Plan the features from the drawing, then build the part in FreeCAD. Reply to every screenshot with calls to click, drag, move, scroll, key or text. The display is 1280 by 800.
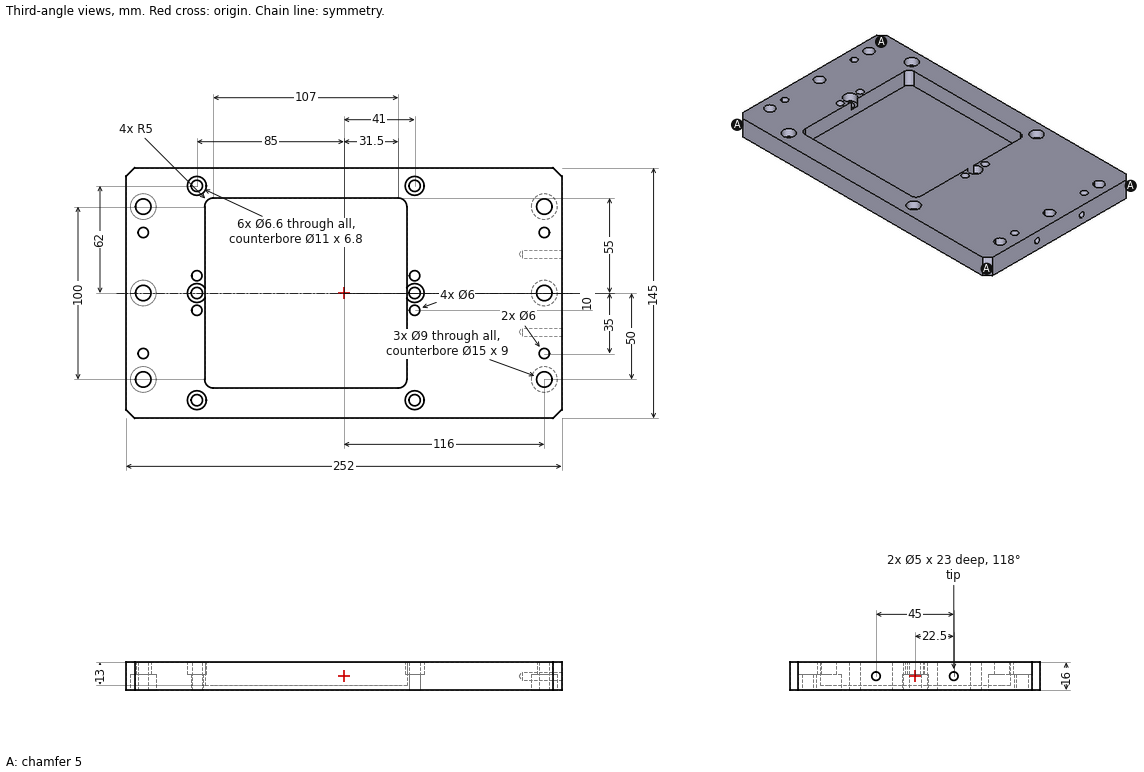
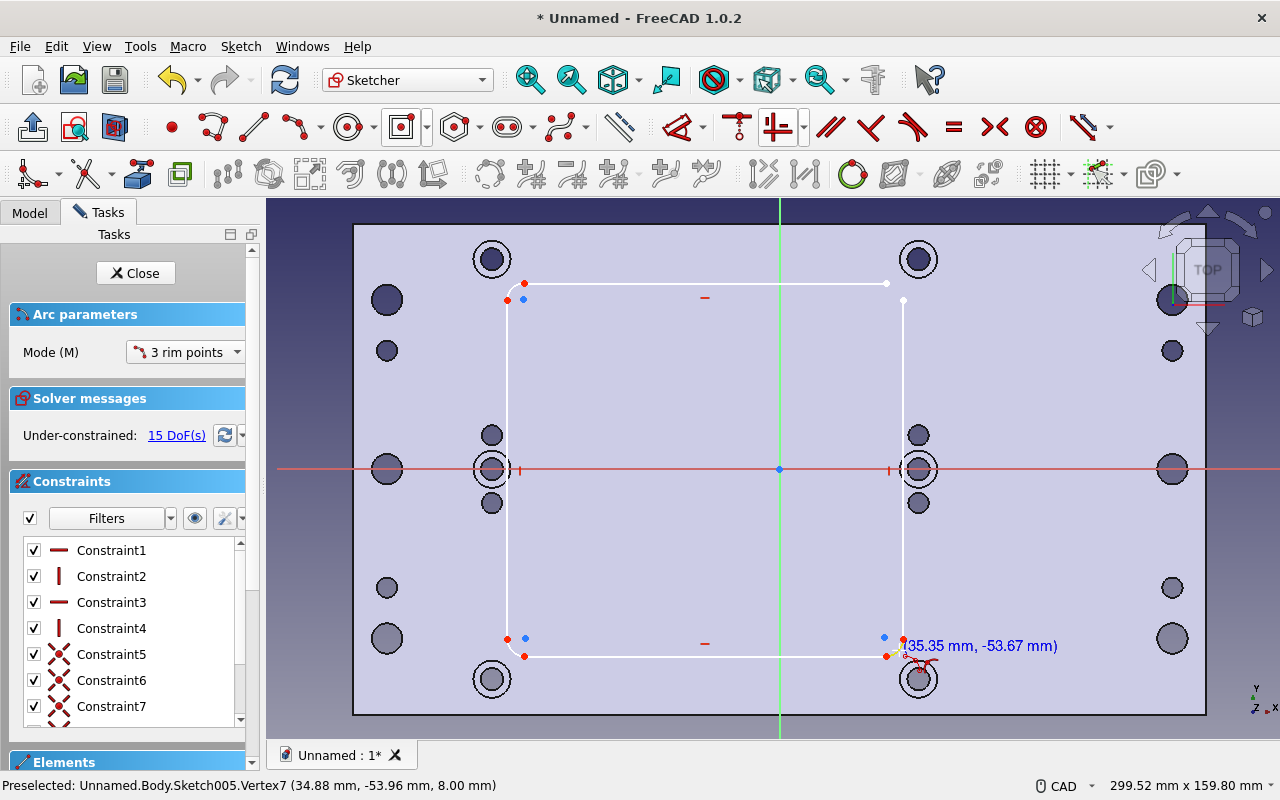
click(903, 301)
click(886, 284)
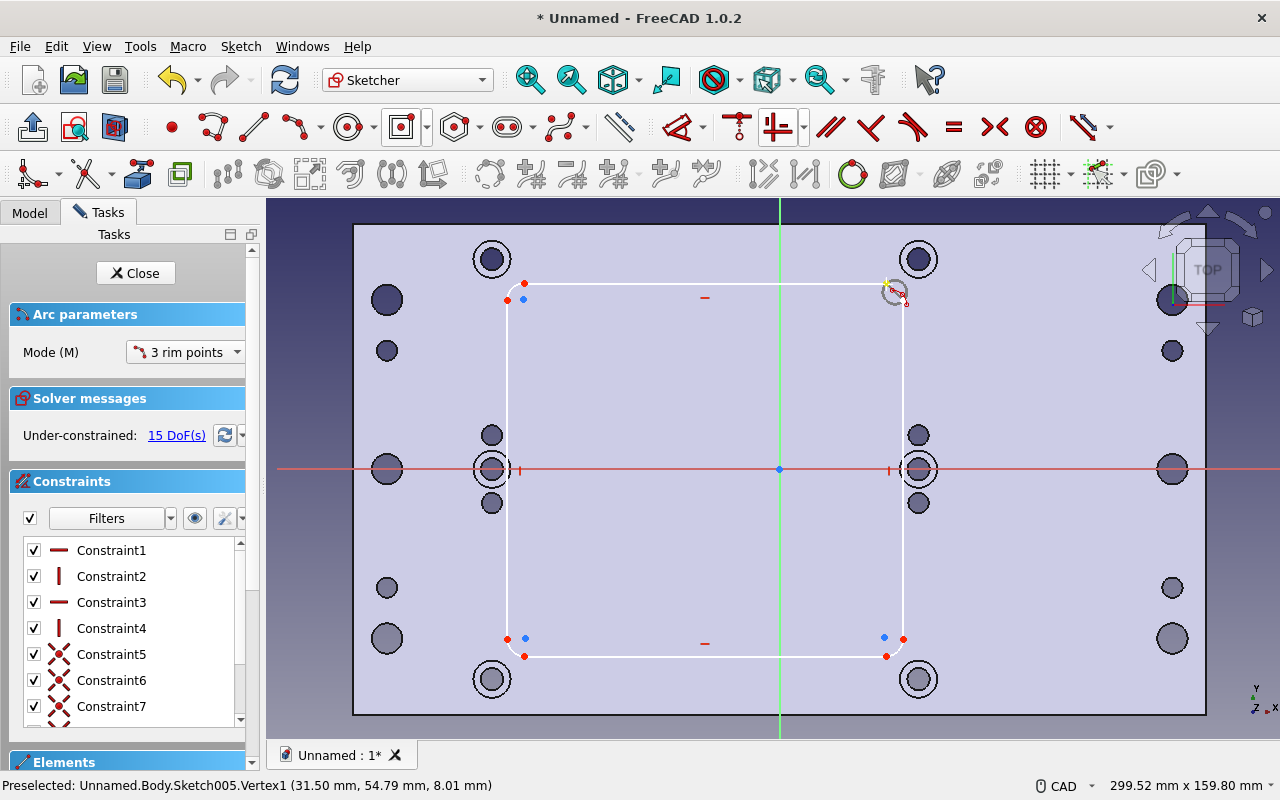
scroll(898, 288, up, 6)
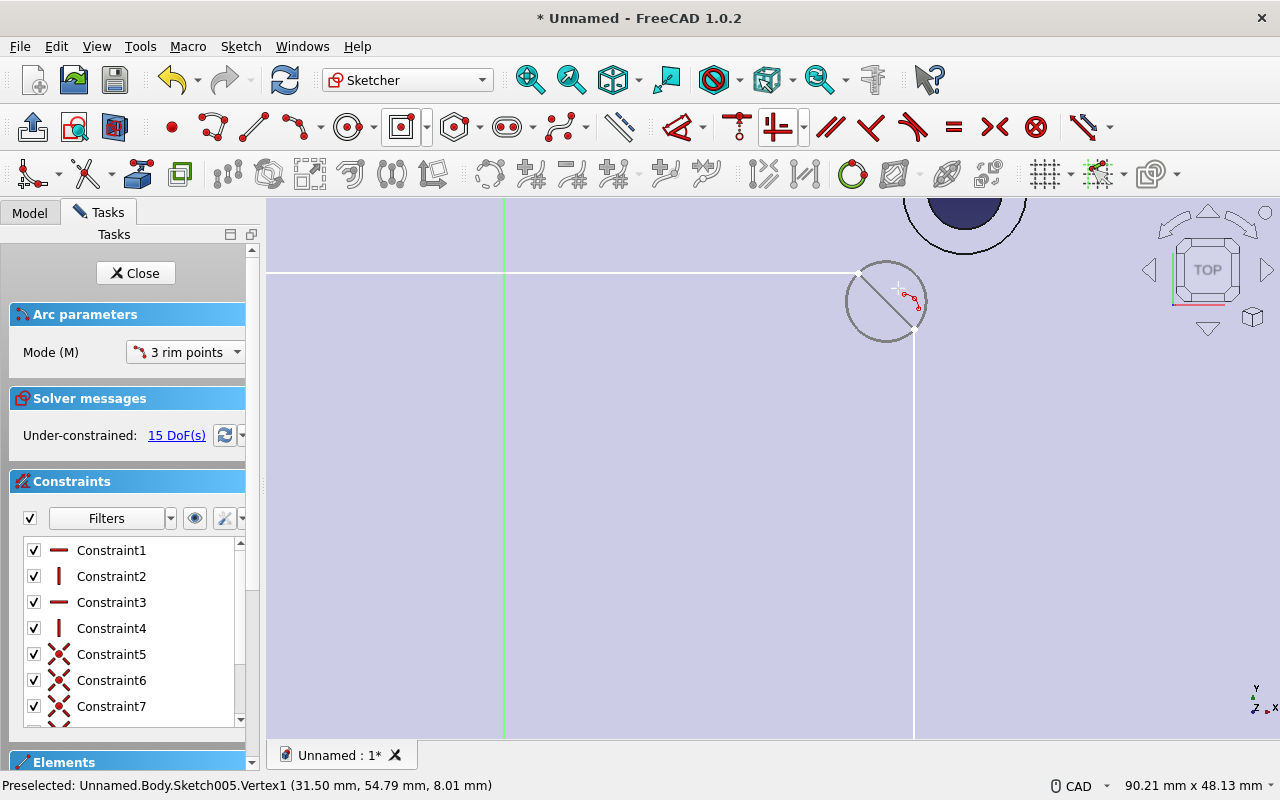
click(898, 287)
key(Escape)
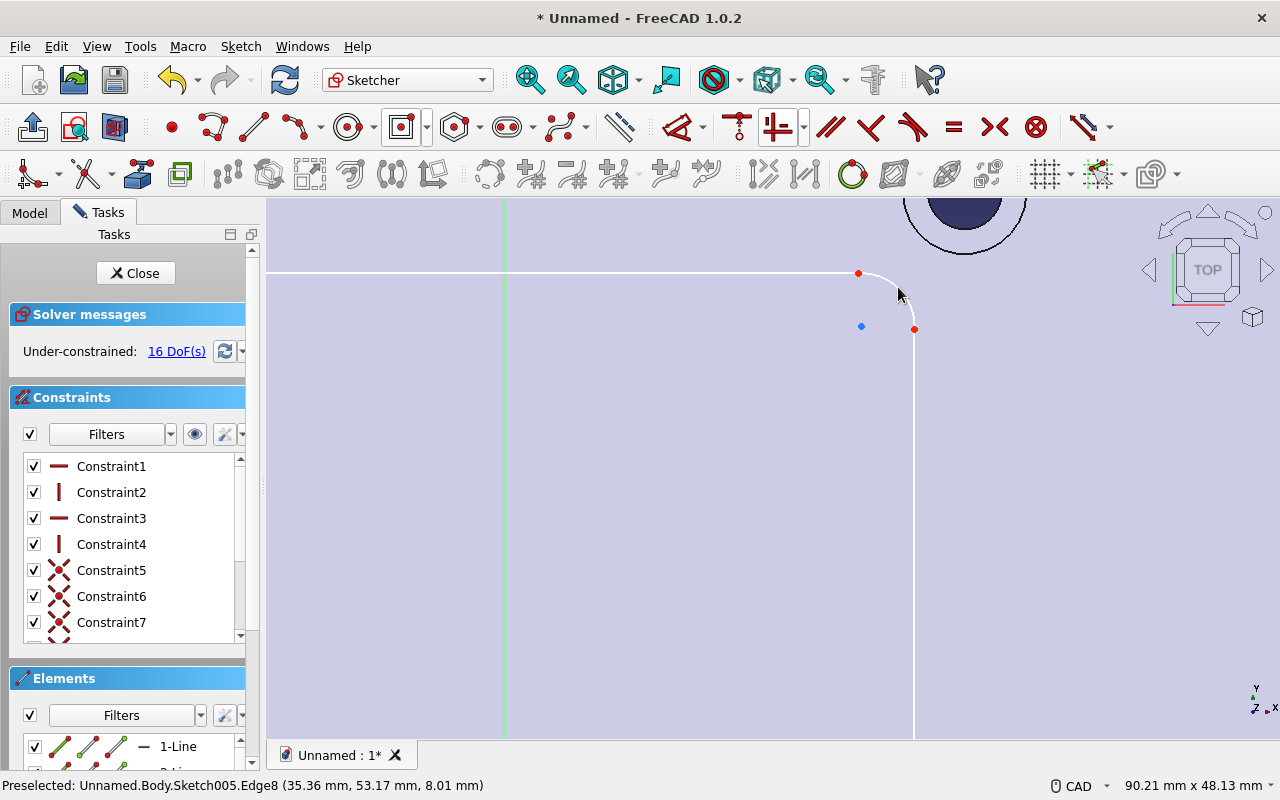
click(377, 273)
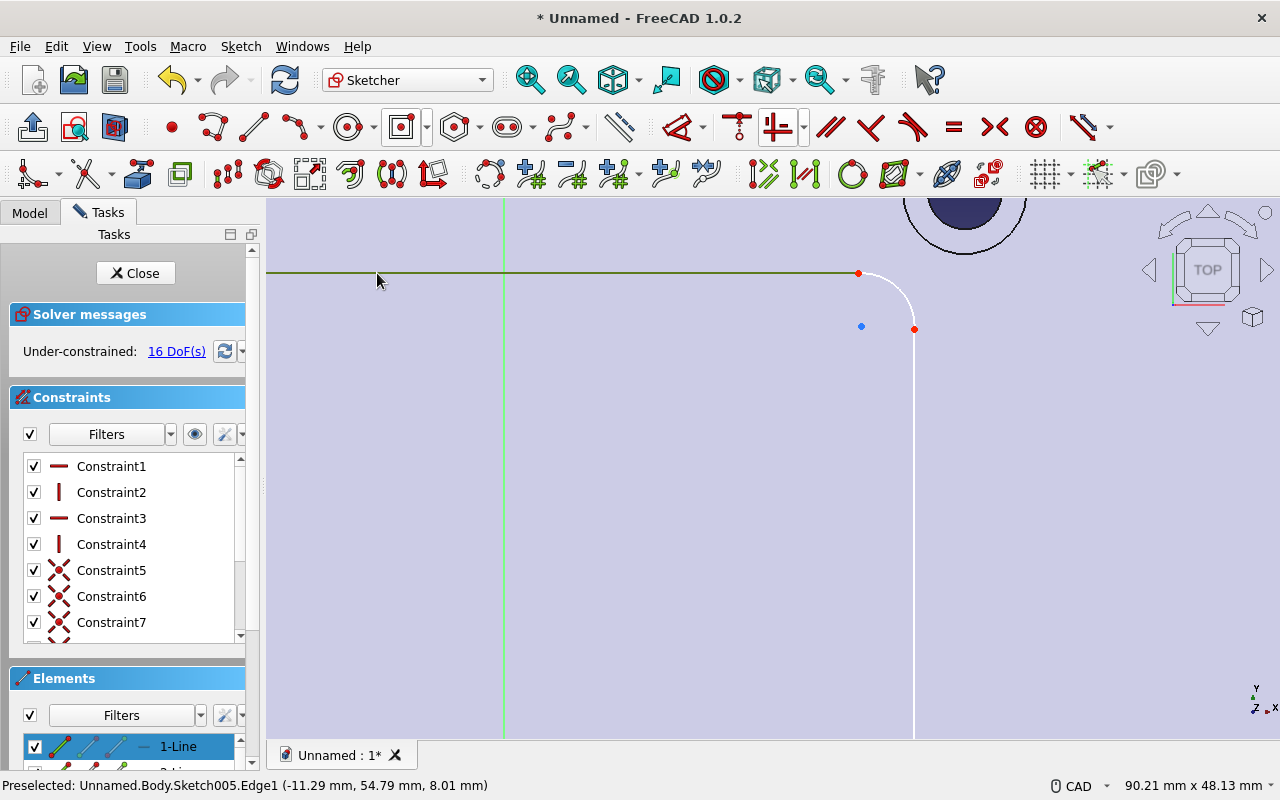
scroll(898, 287, down, 6)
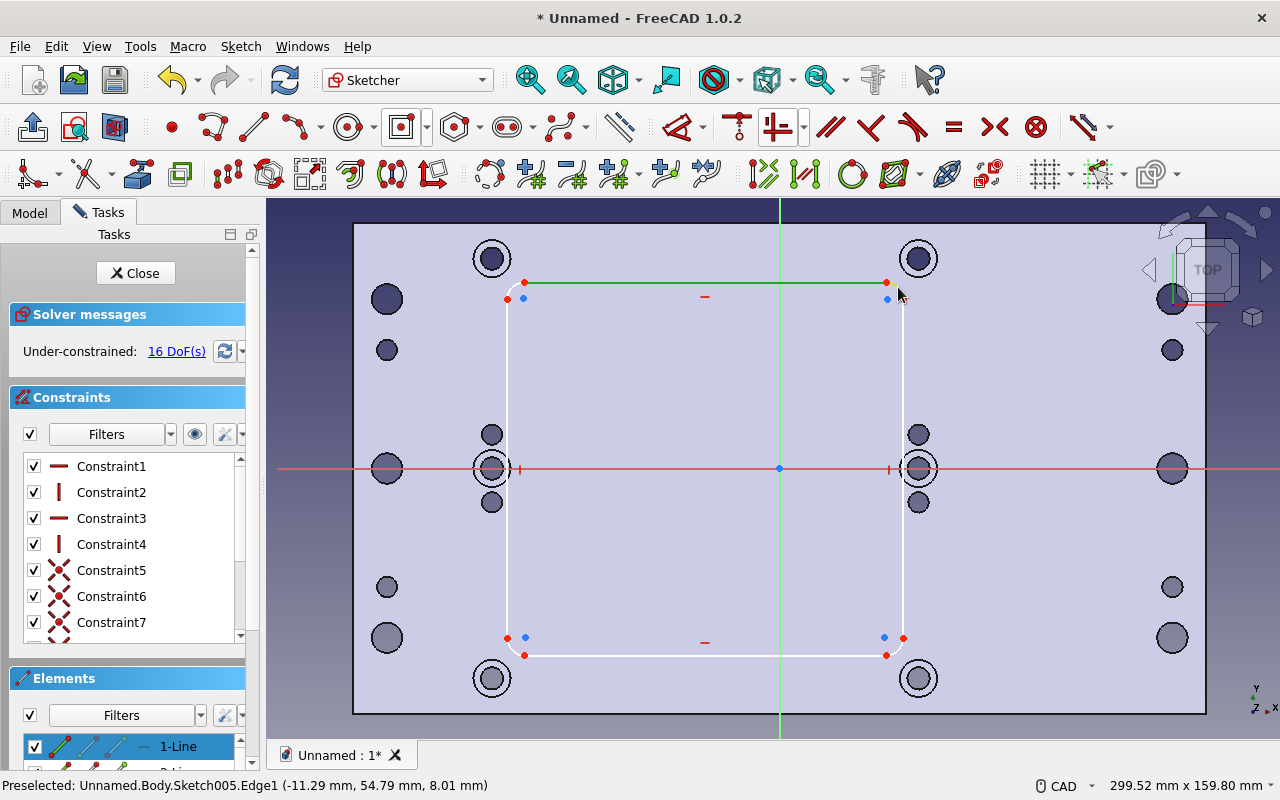
scroll(516, 285, up, 3)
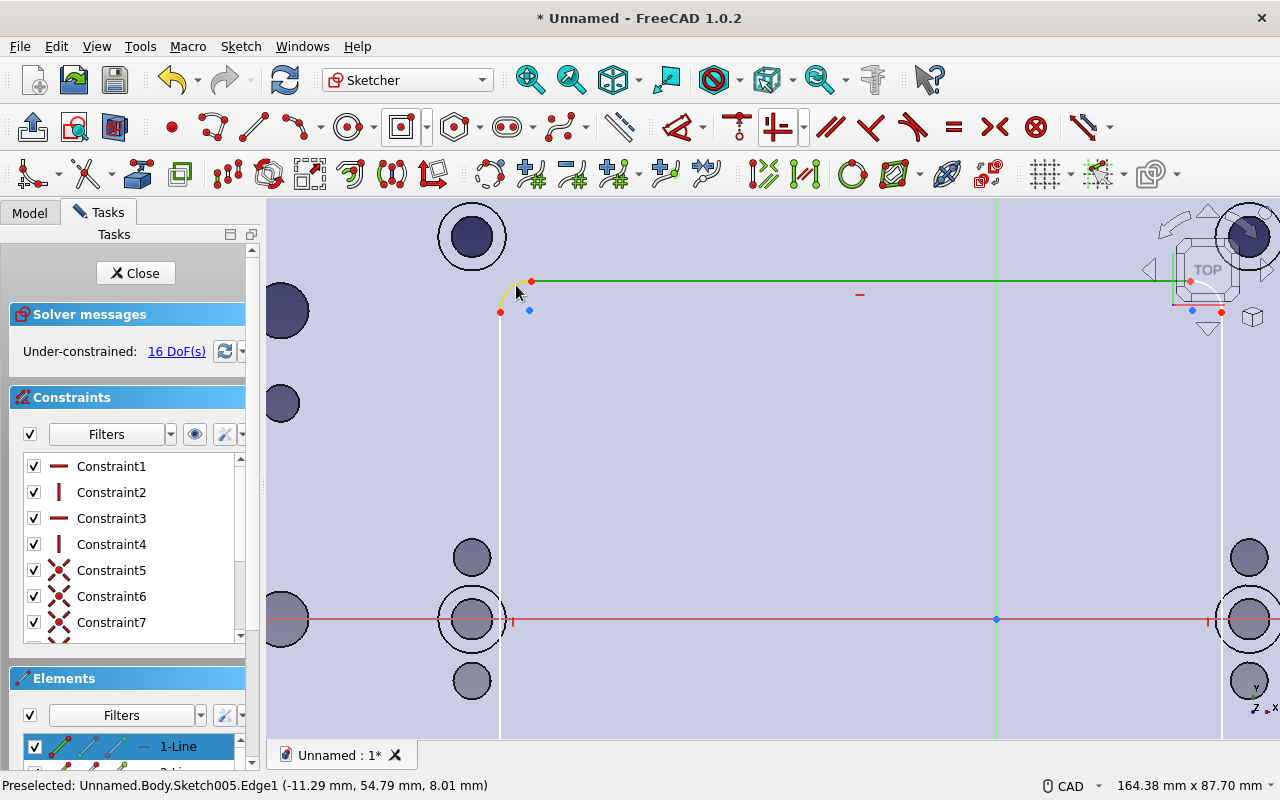
click(517, 284)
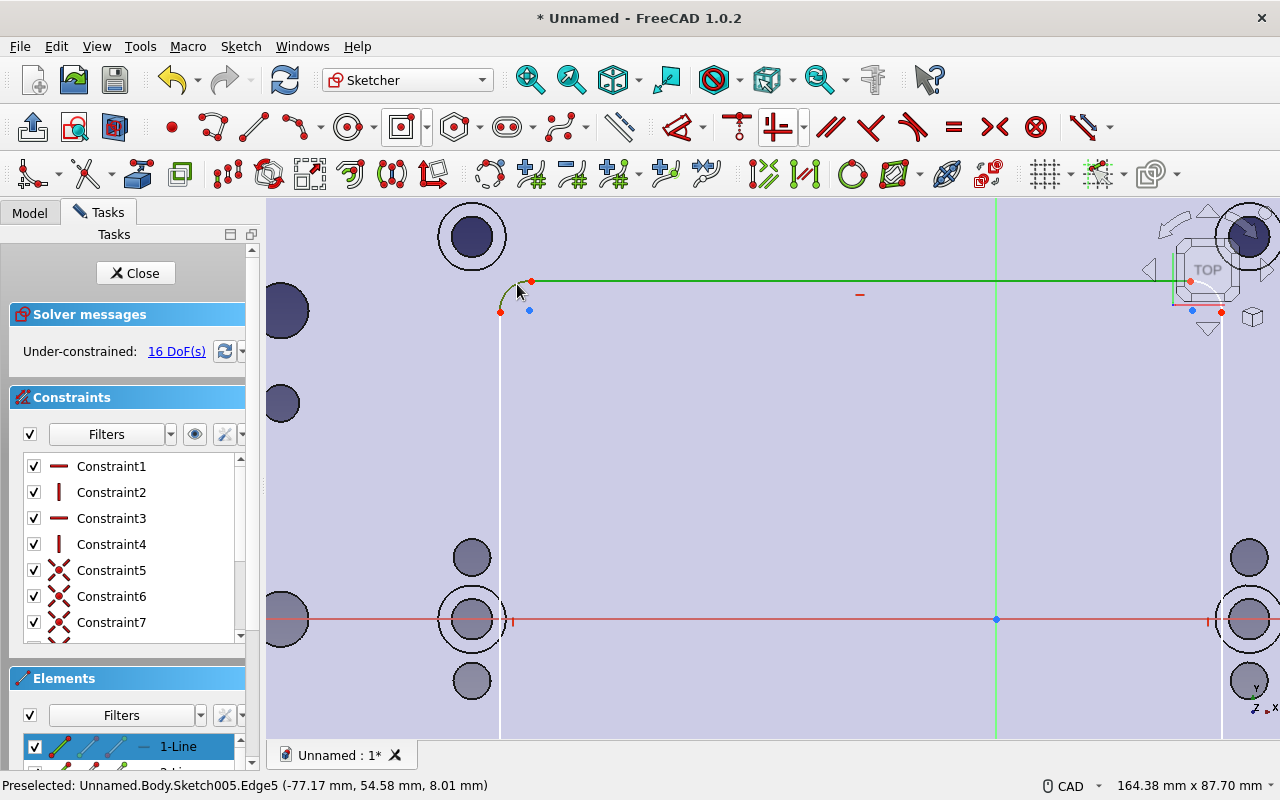
click(913, 128)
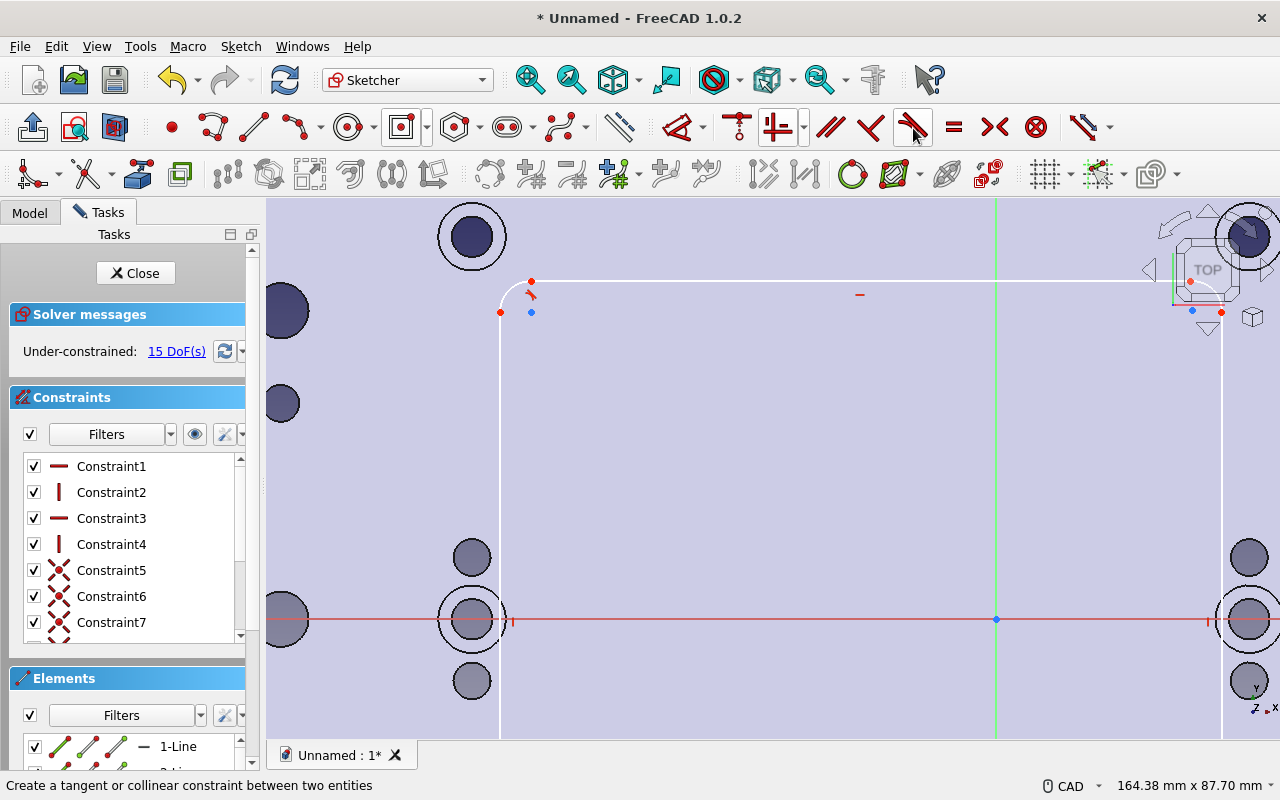
click(993, 281)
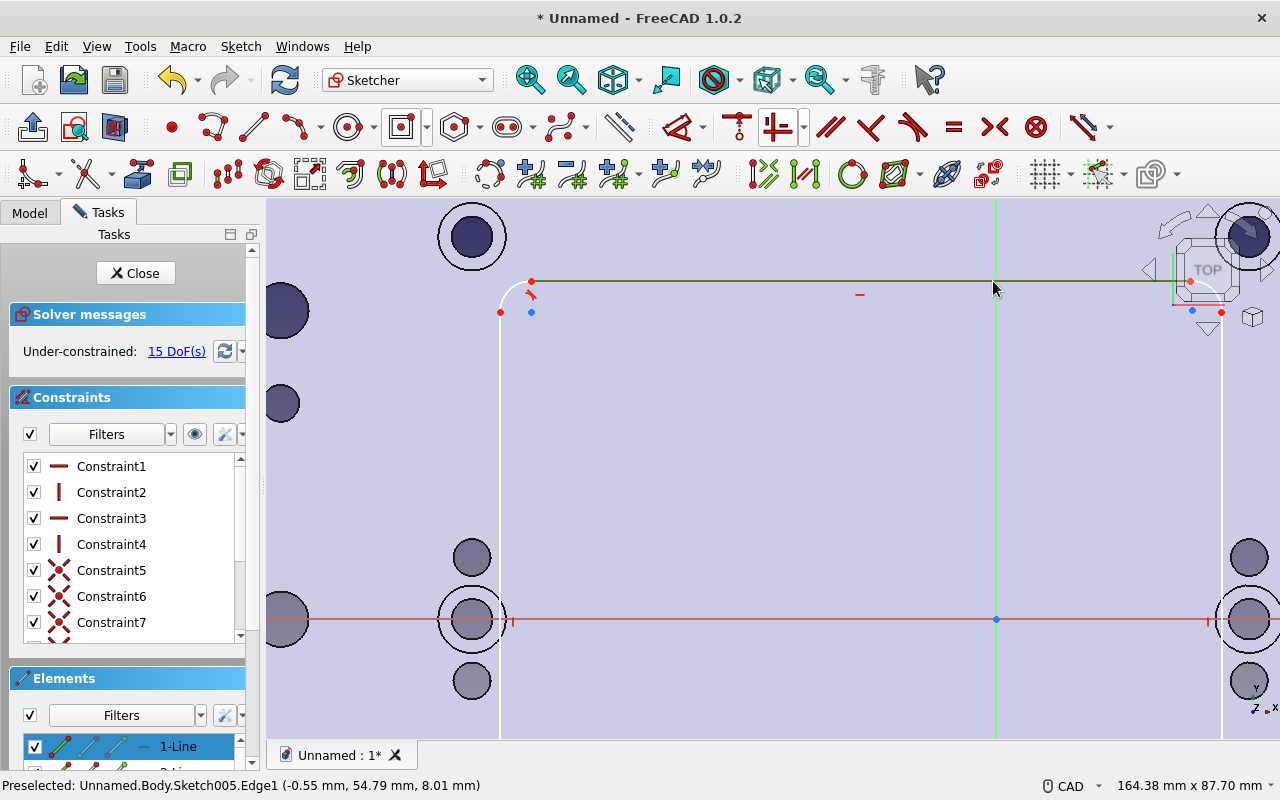
scroll(515, 285, down, 3)